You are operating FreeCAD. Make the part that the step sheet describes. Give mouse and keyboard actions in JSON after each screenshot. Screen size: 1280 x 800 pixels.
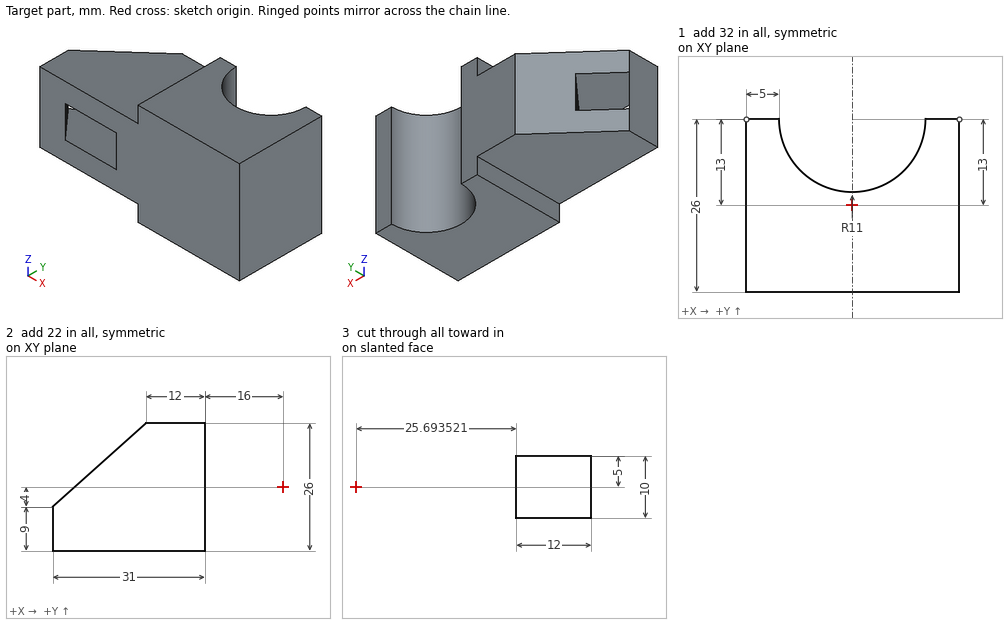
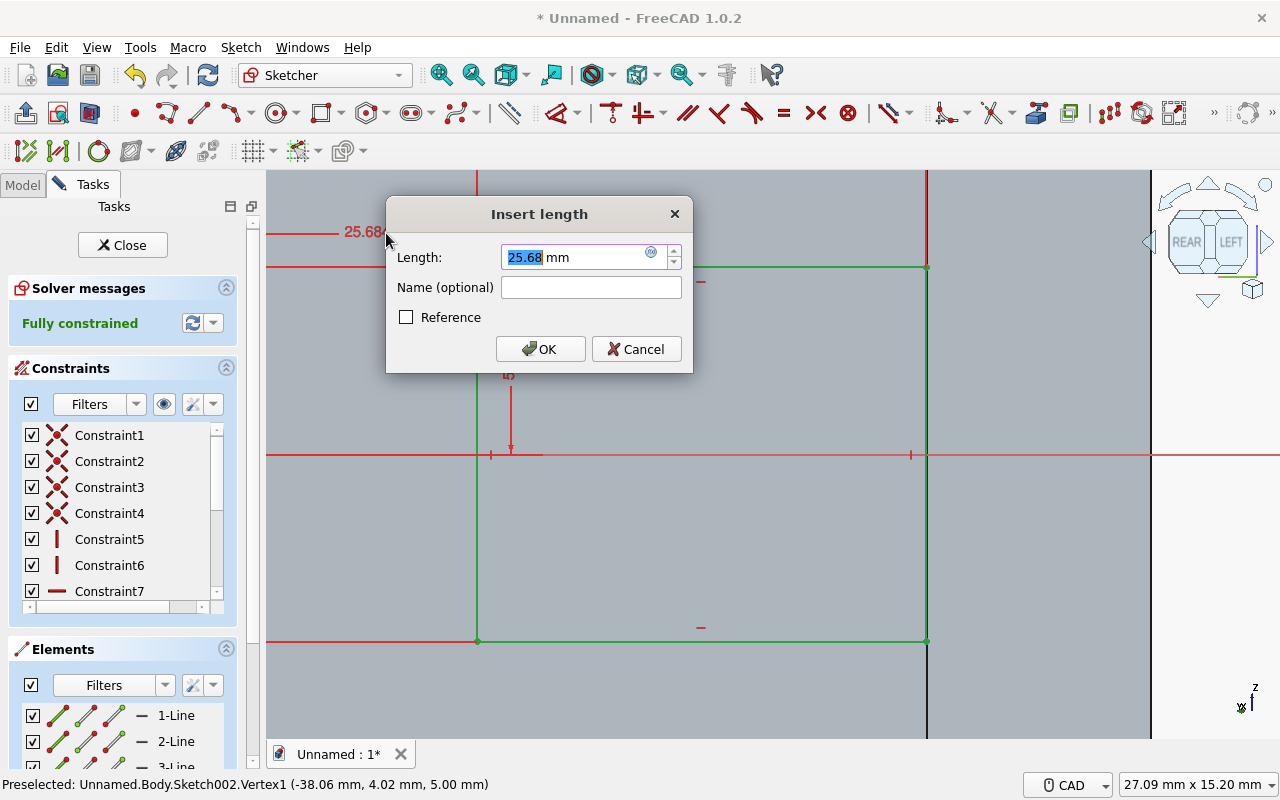
{"action": "type", "text": "25.693521"}
{"action": "key", "text": "Return"}
{"action": "key", "text": "Escape"}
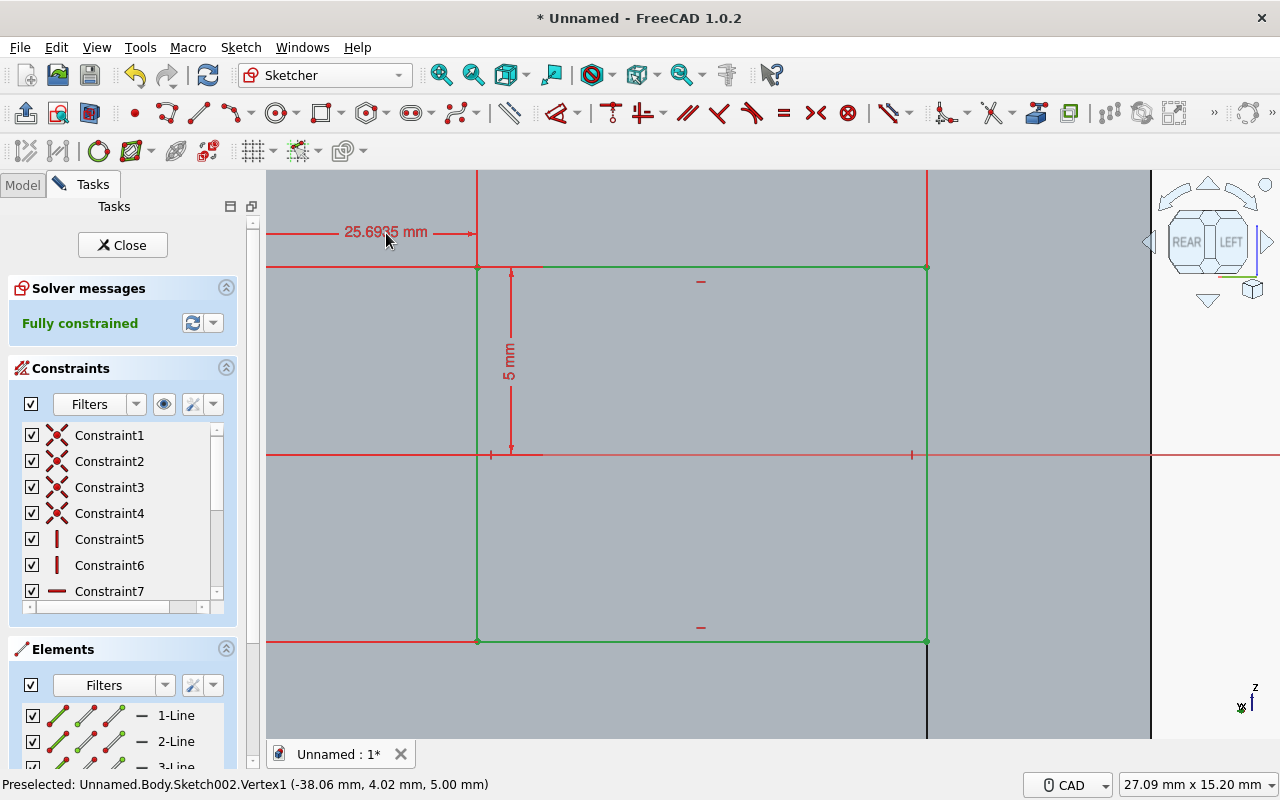
{"action": "left_click", "coordinate": [123, 245]}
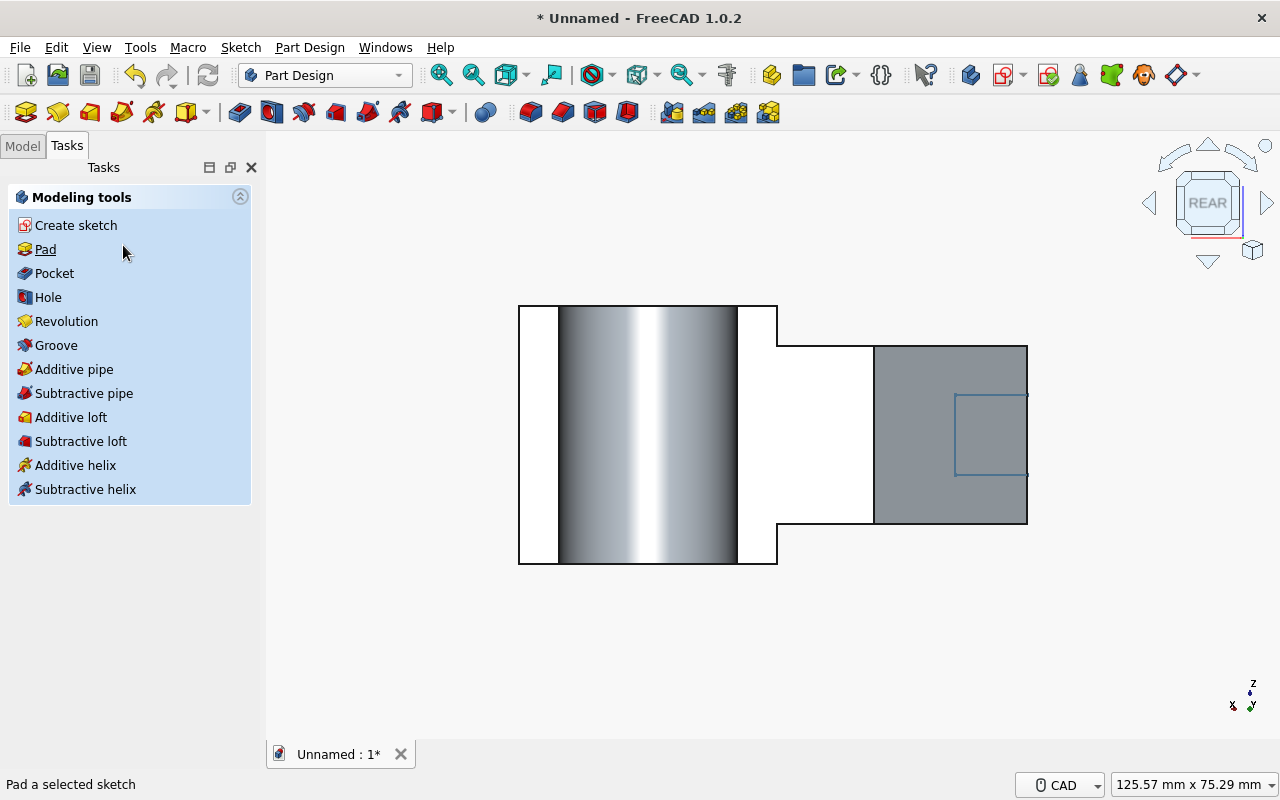
{"action": "left_click", "coordinate": [240, 112]}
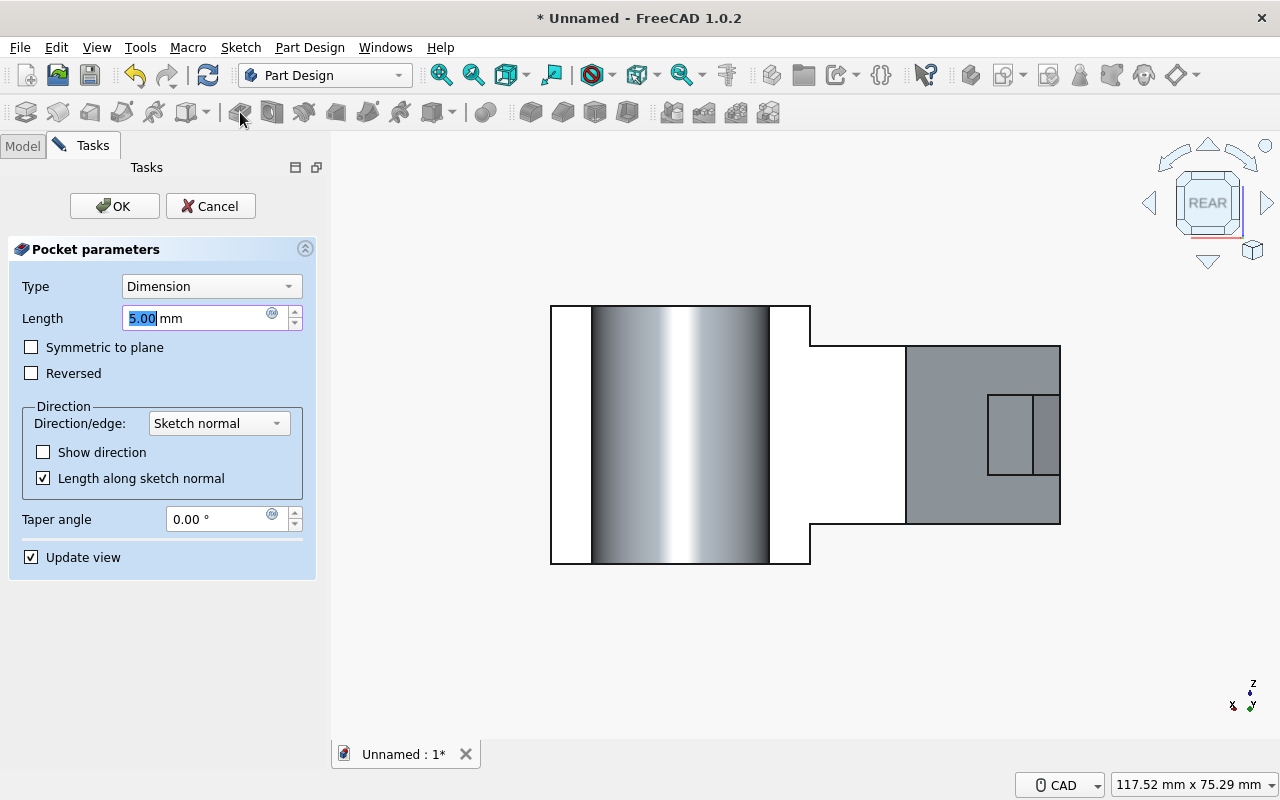
{"action": "left_click", "coordinate": [212, 286]}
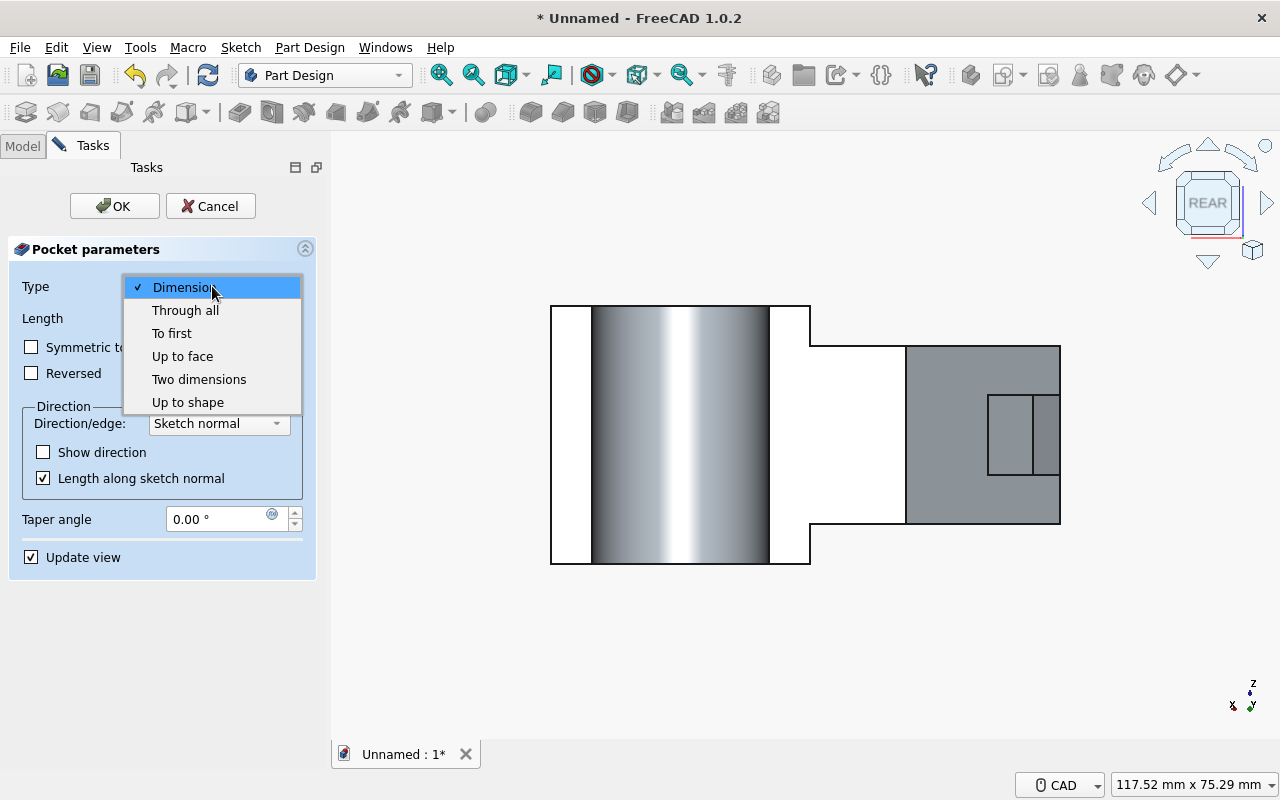
{"action": "left_click", "coordinate": [212, 310]}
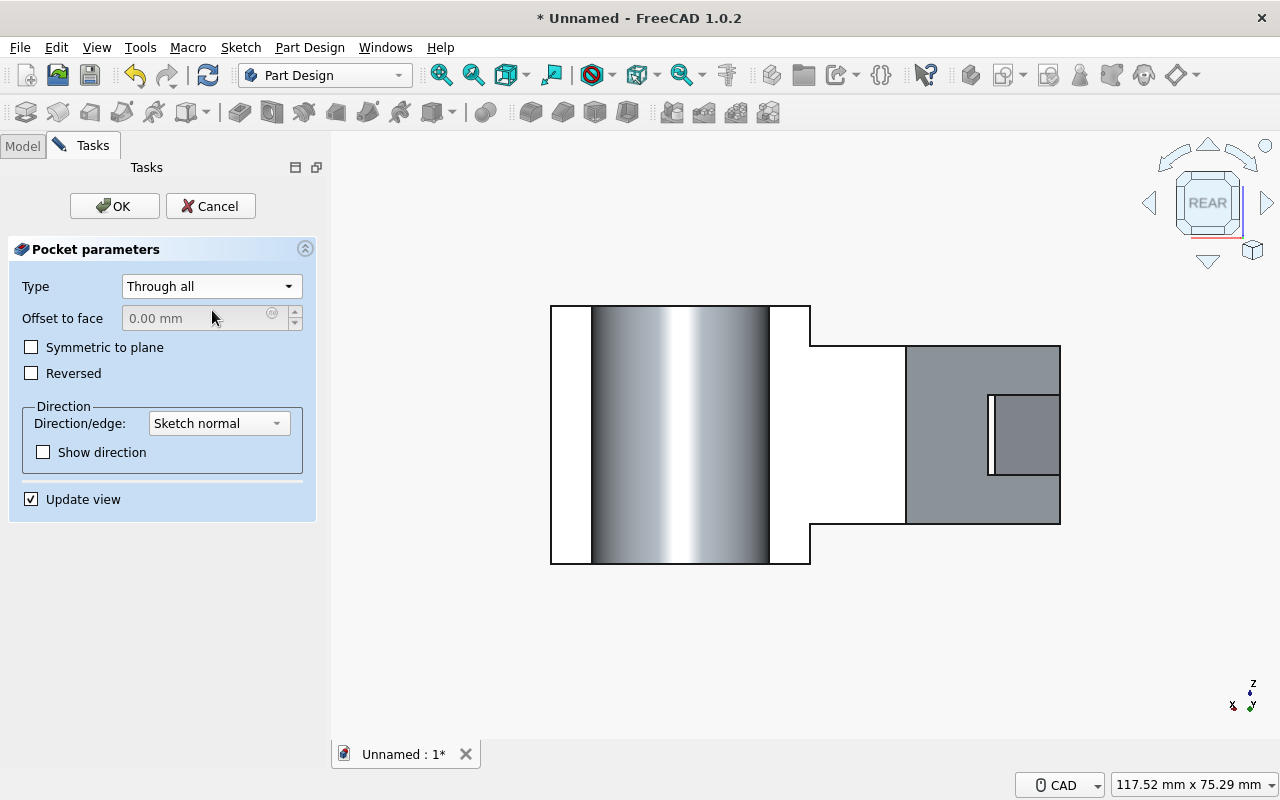
{"action": "left_click", "coordinate": [115, 206]}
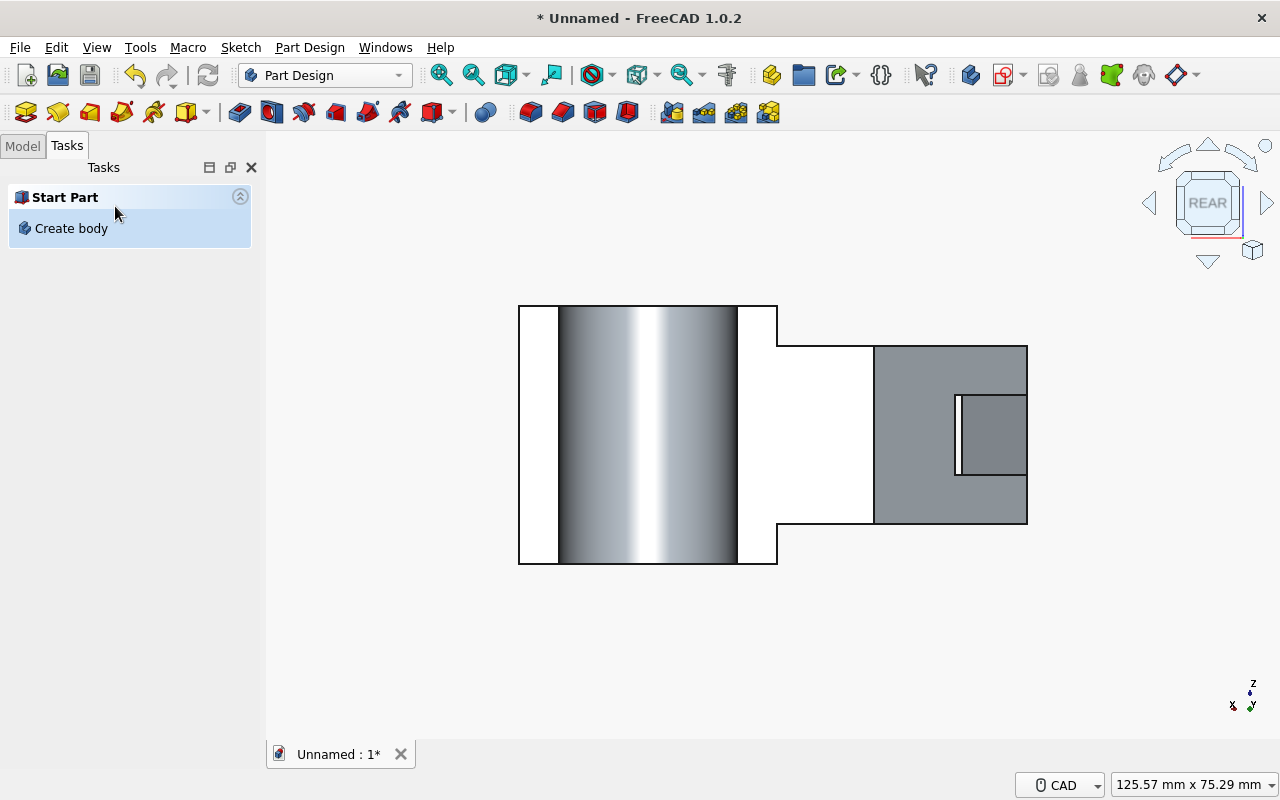
{"action": "key", "text": "0"}